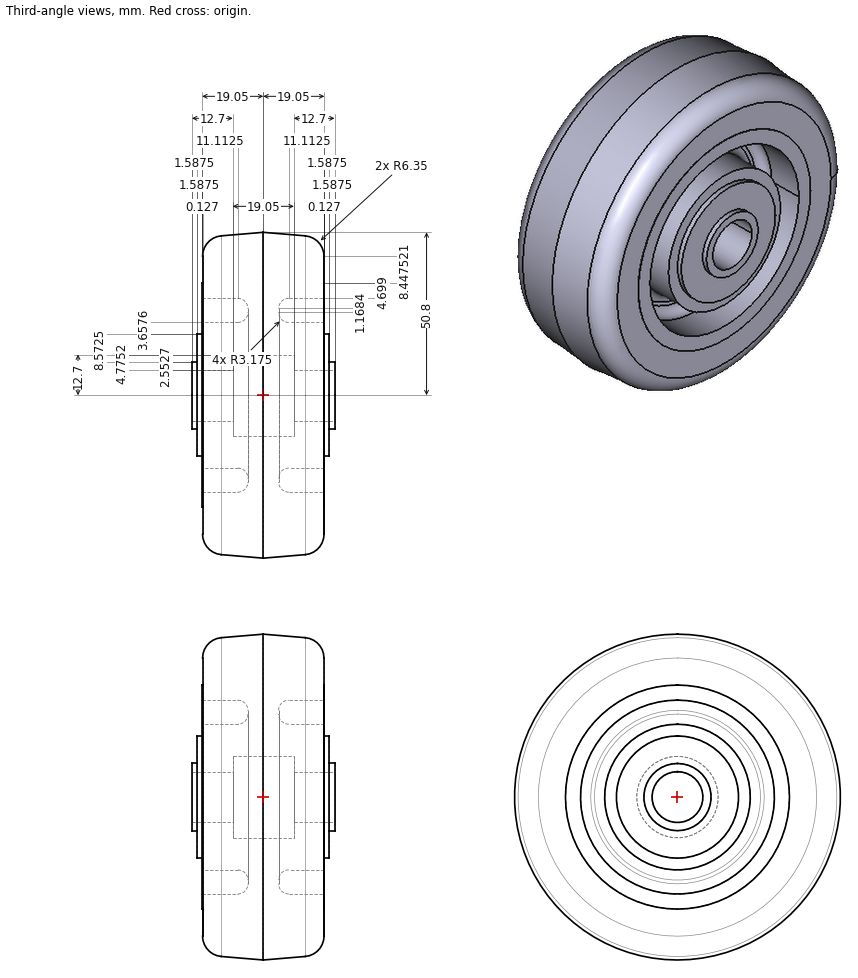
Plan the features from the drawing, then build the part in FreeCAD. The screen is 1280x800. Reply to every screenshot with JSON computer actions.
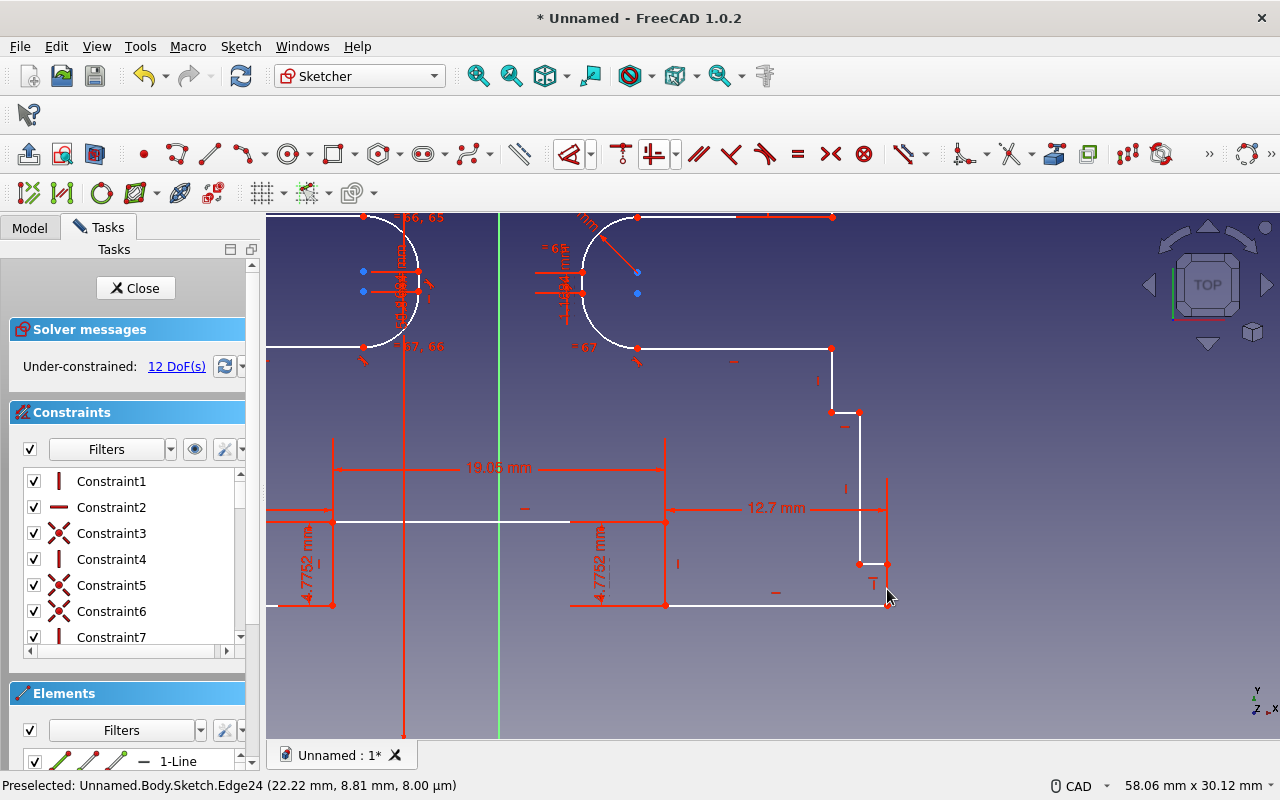
{"action": "left_click", "coordinate": [590, 154]}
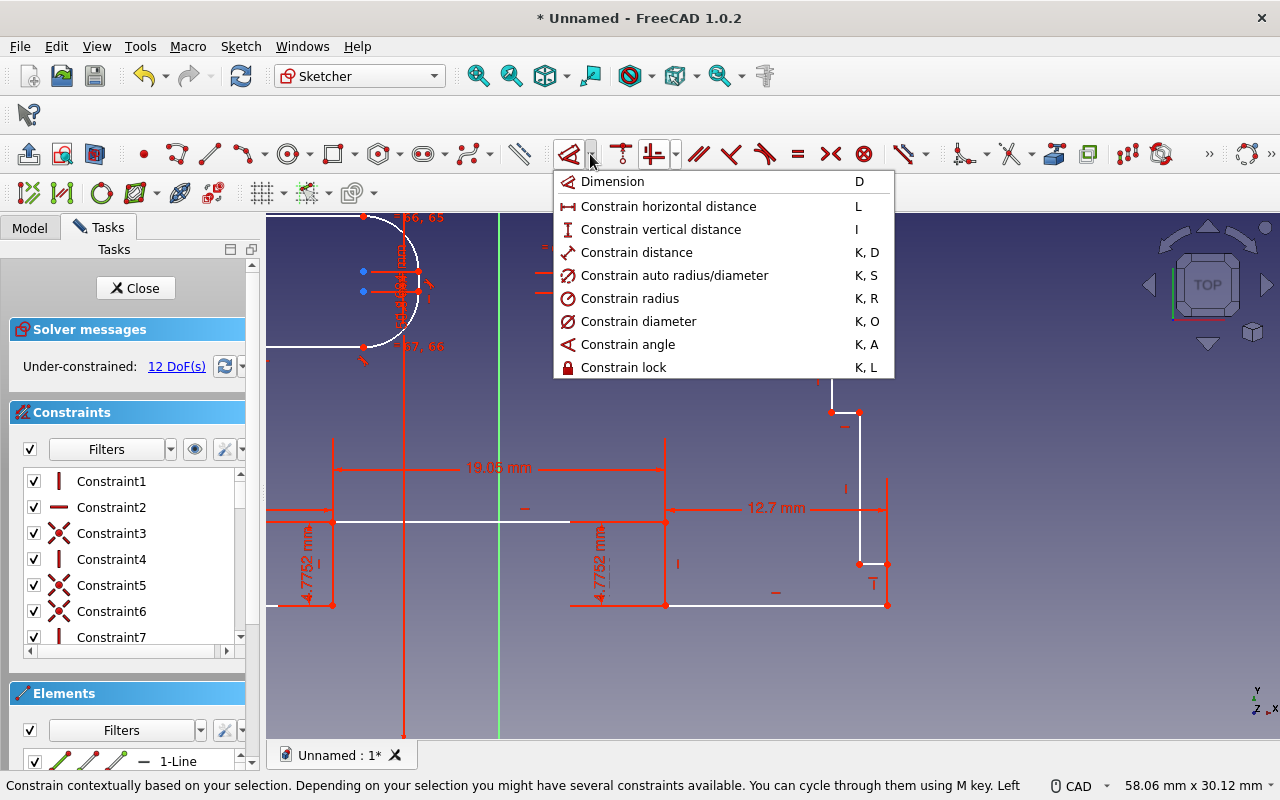
{"action": "left_click", "coordinate": [724, 230]}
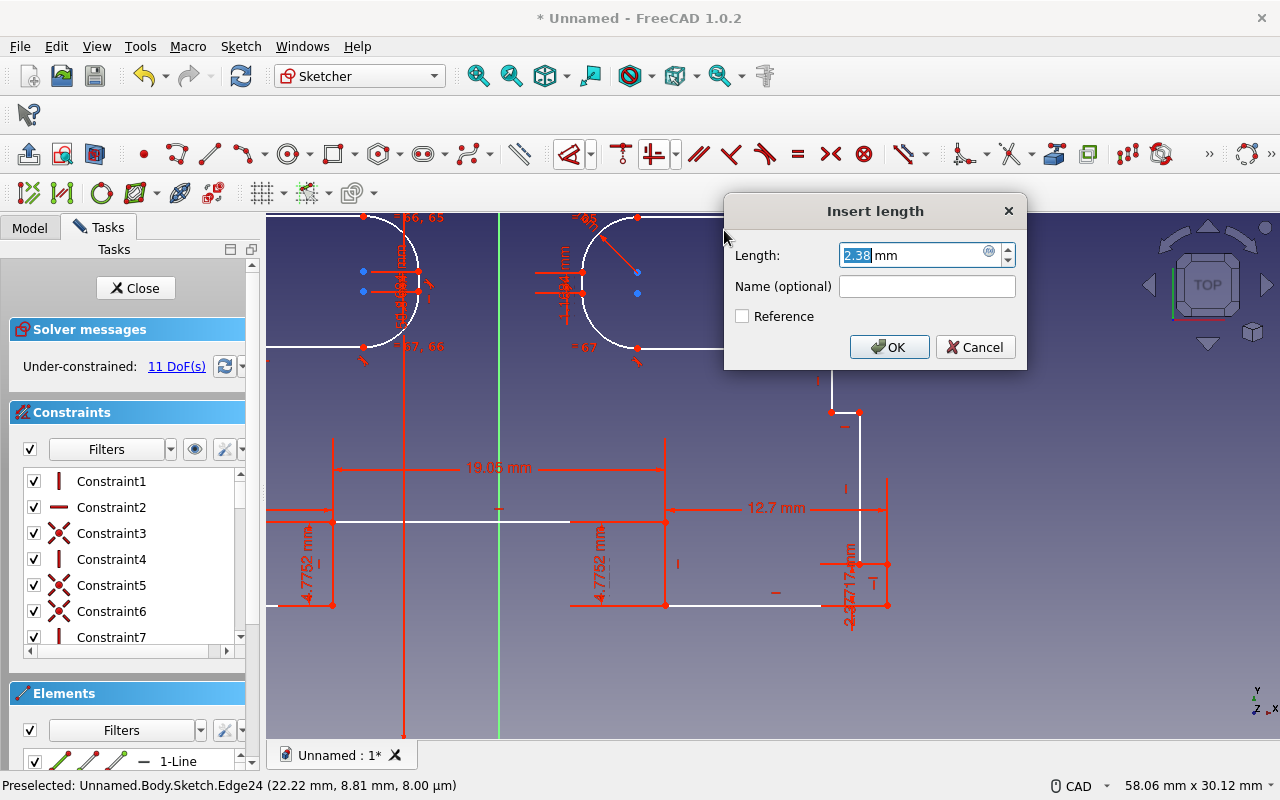
{"action": "type", "text": "2.5527"}
{"action": "key", "text": "Return"}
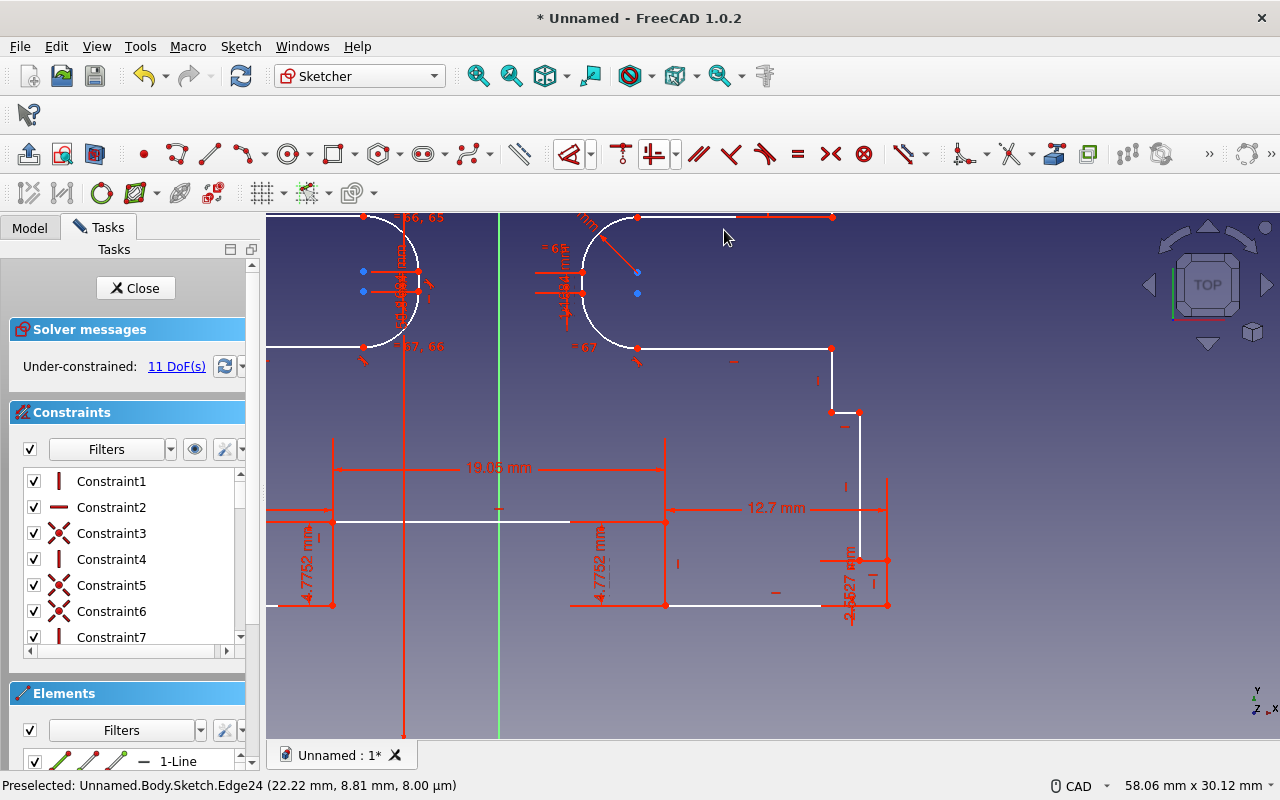
{"action": "scroll", "coordinate": [876, 561], "scroll_direction": "up", "scroll_amount": 2}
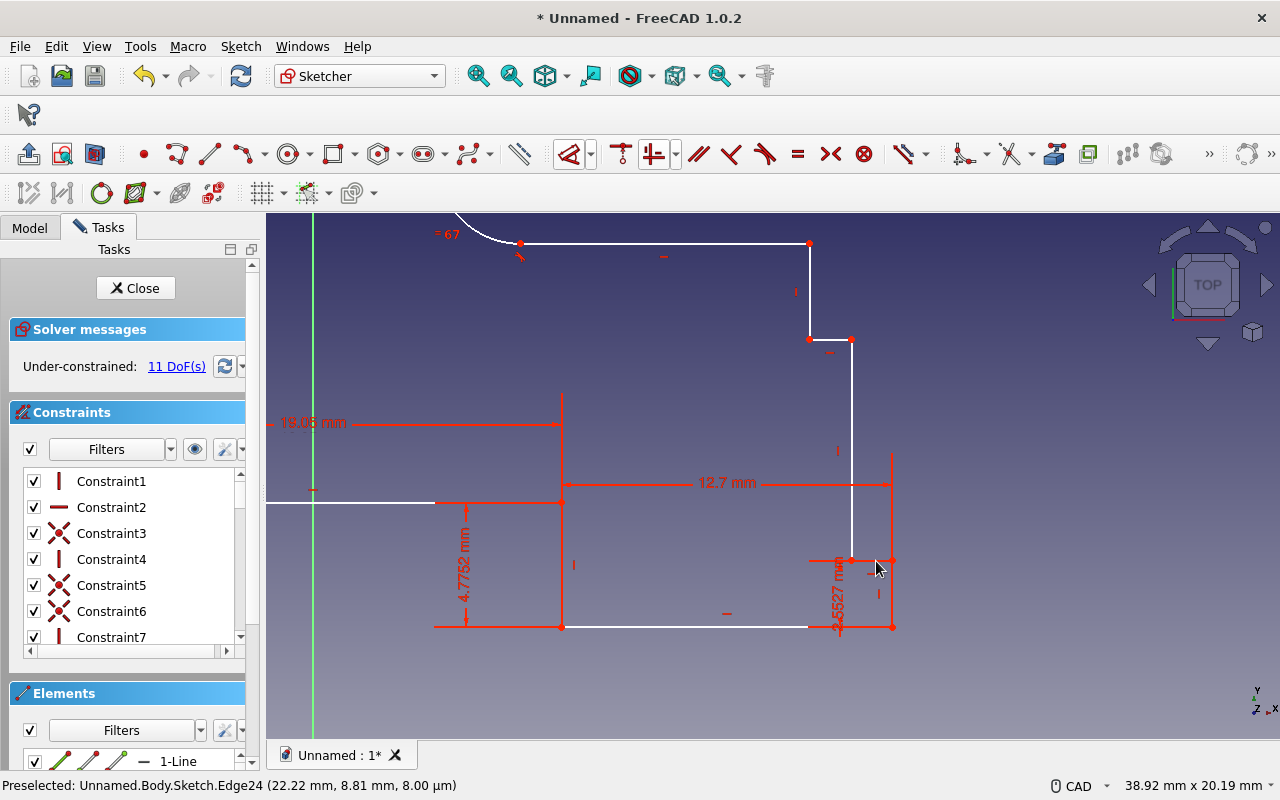
{"action": "left_click", "coordinate": [876, 561]}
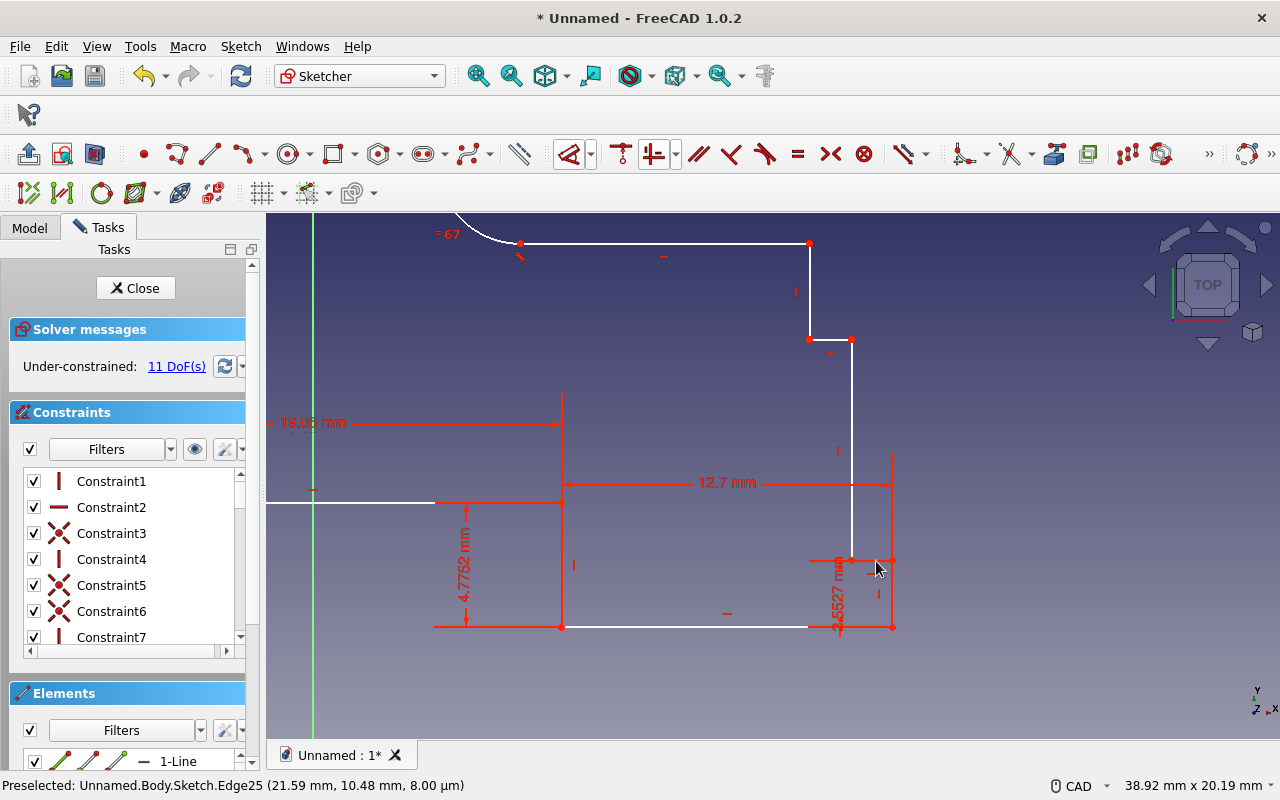
{"action": "left_click", "coordinate": [590, 154]}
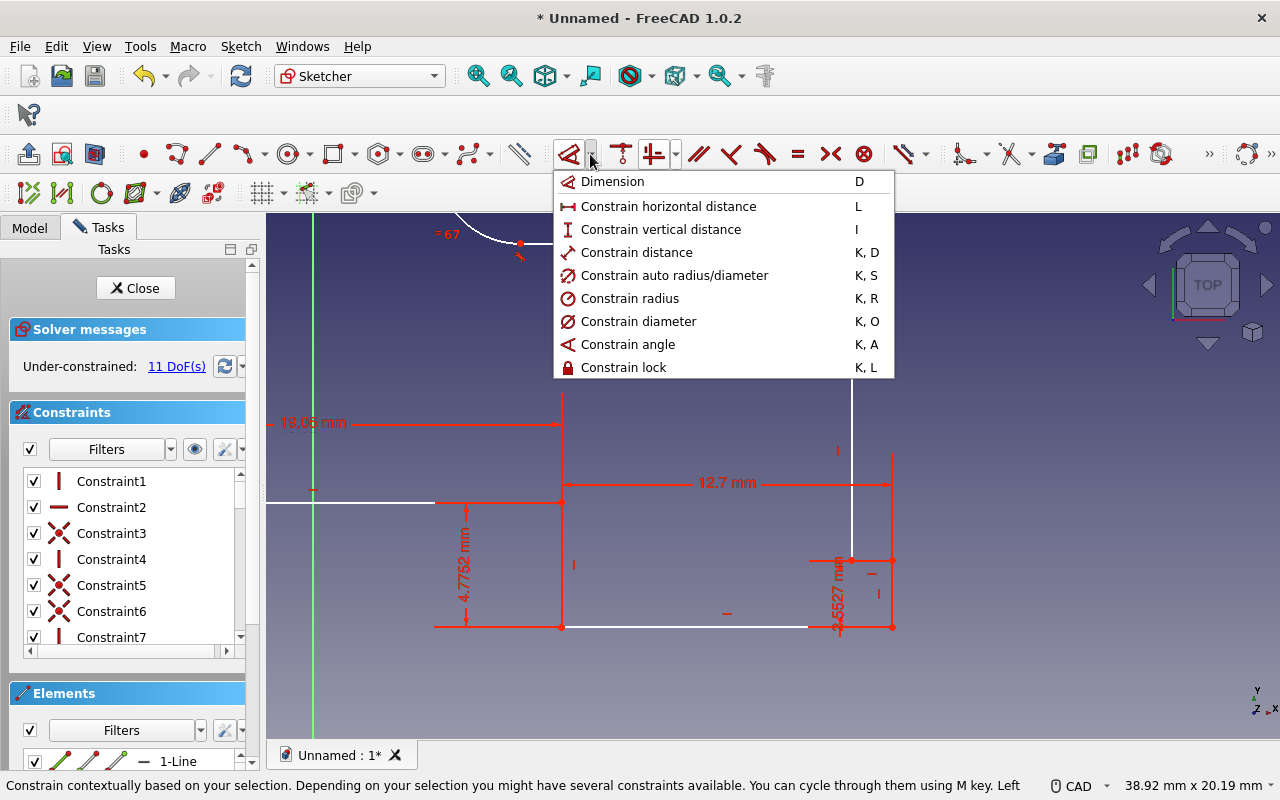
{"action": "left_click", "coordinate": [724, 206]}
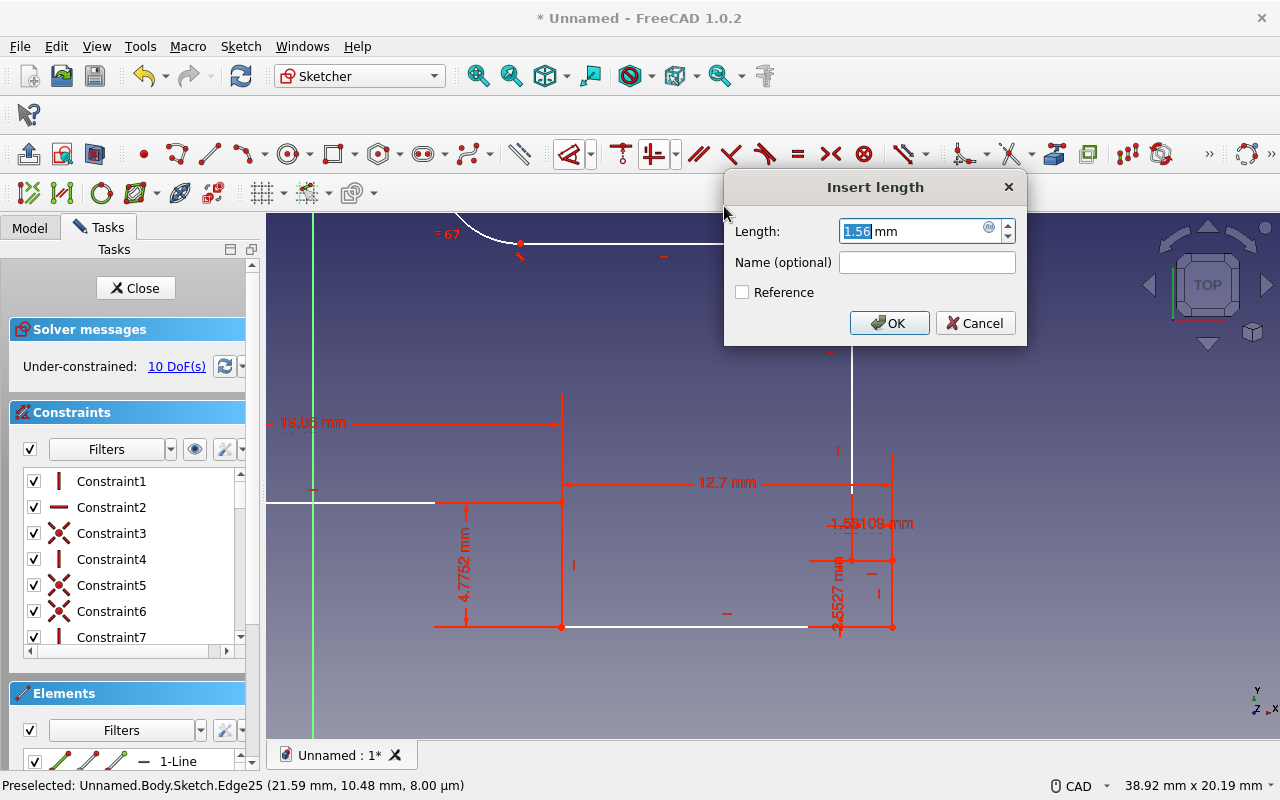
{"action": "type", "text": "1.5875"}
{"action": "key", "text": "Return"}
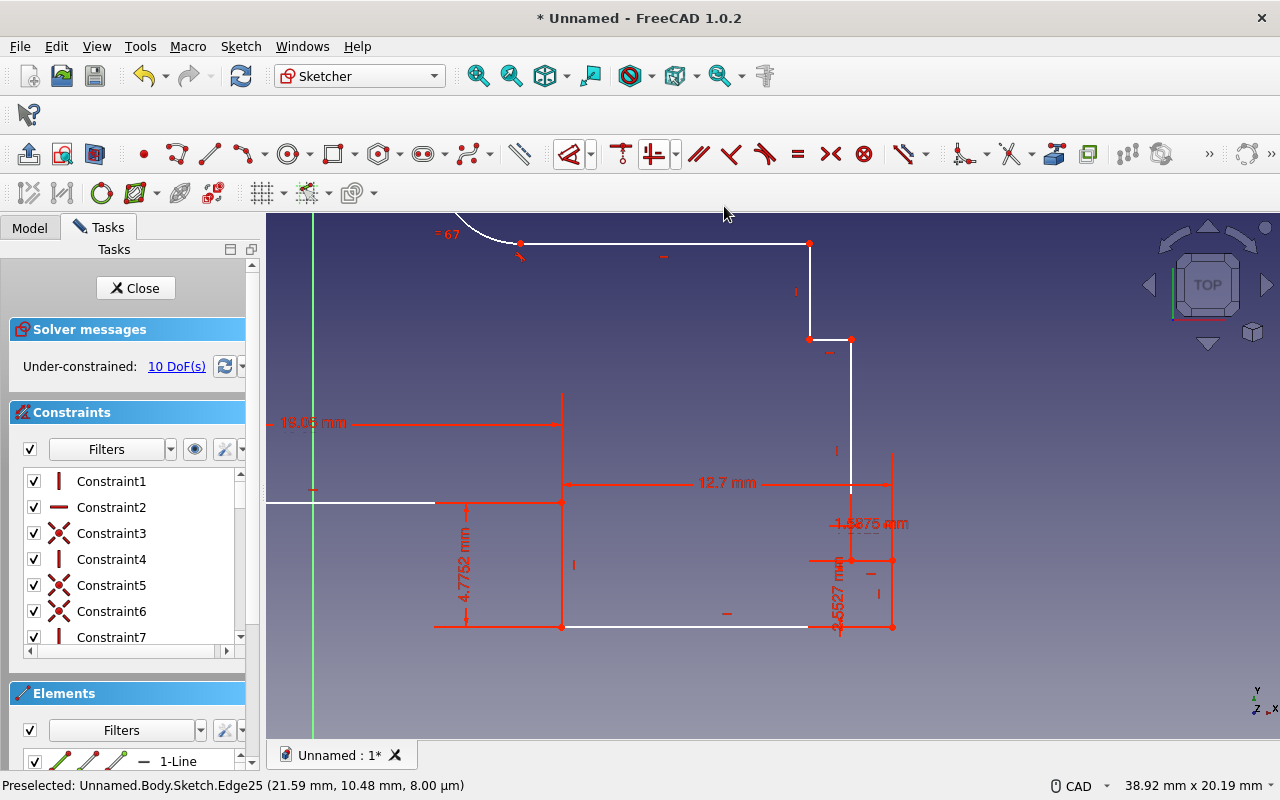
{"action": "scroll", "coordinate": [832, 576], "scroll_direction": "down", "scroll_amount": 7}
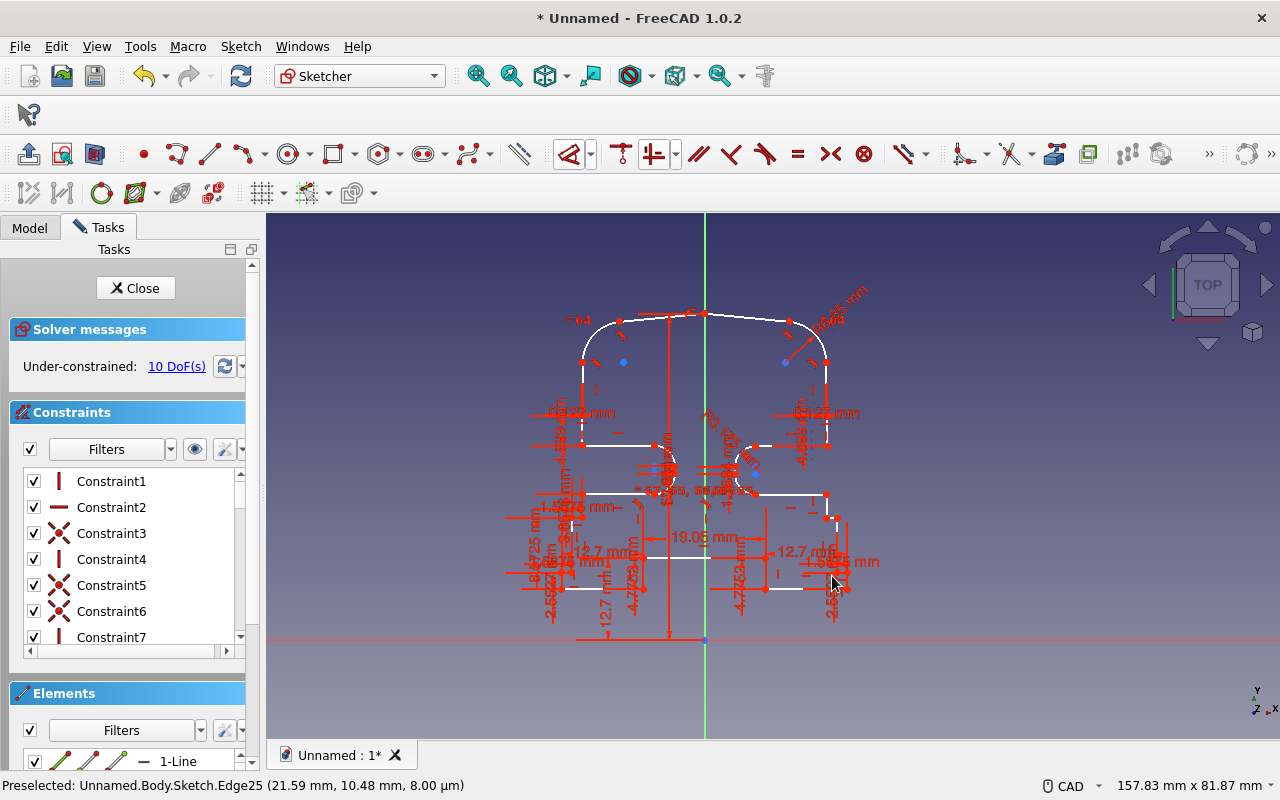
{"action": "left_click", "coordinate": [837, 535]}